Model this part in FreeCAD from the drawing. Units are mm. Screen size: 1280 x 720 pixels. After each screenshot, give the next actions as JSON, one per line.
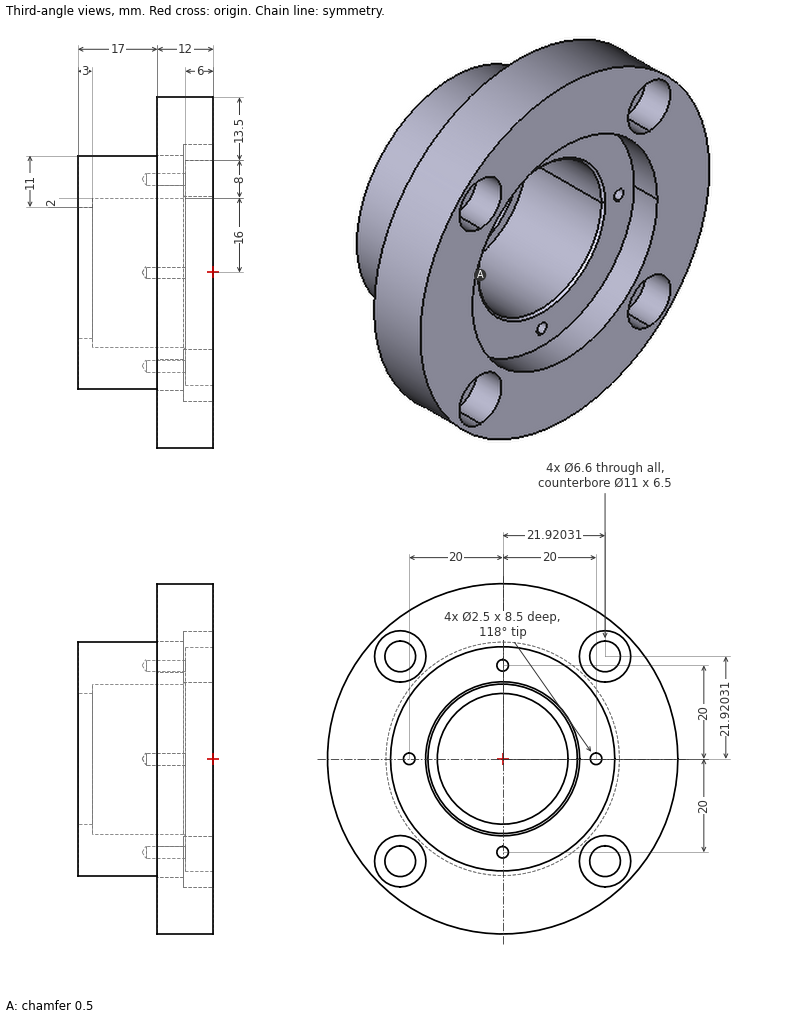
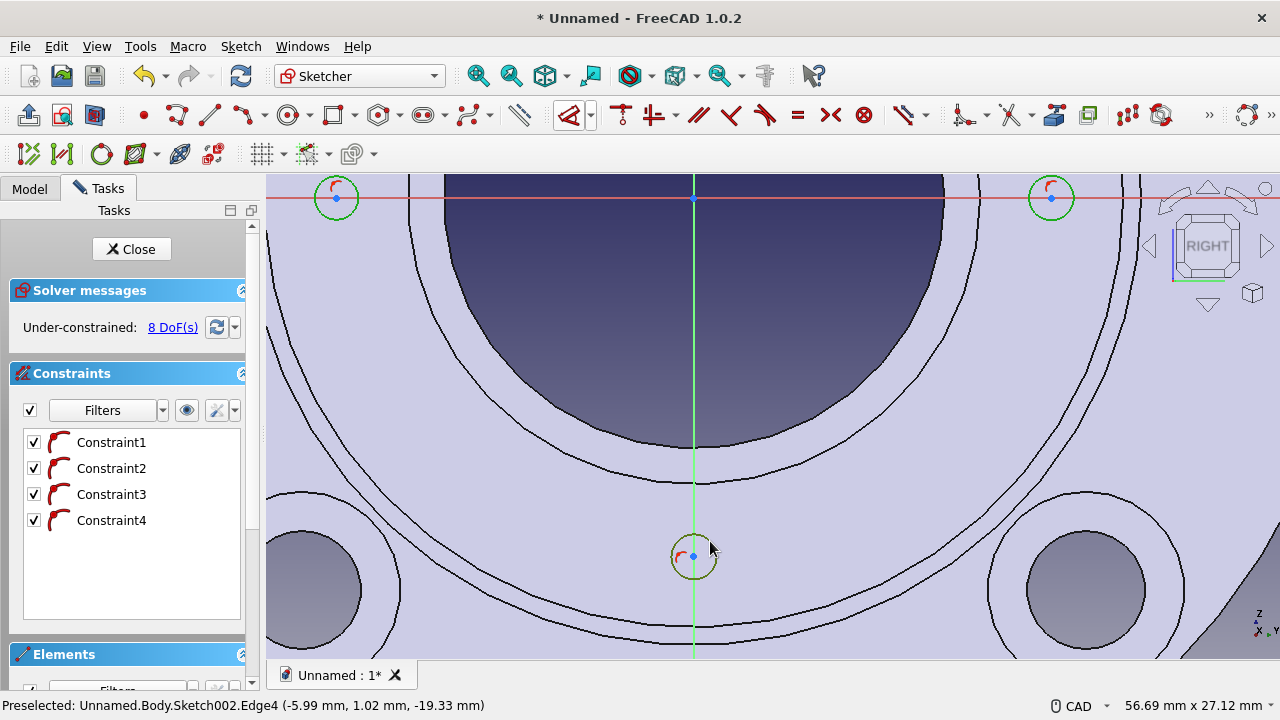
{"action": "key", "text": "e"}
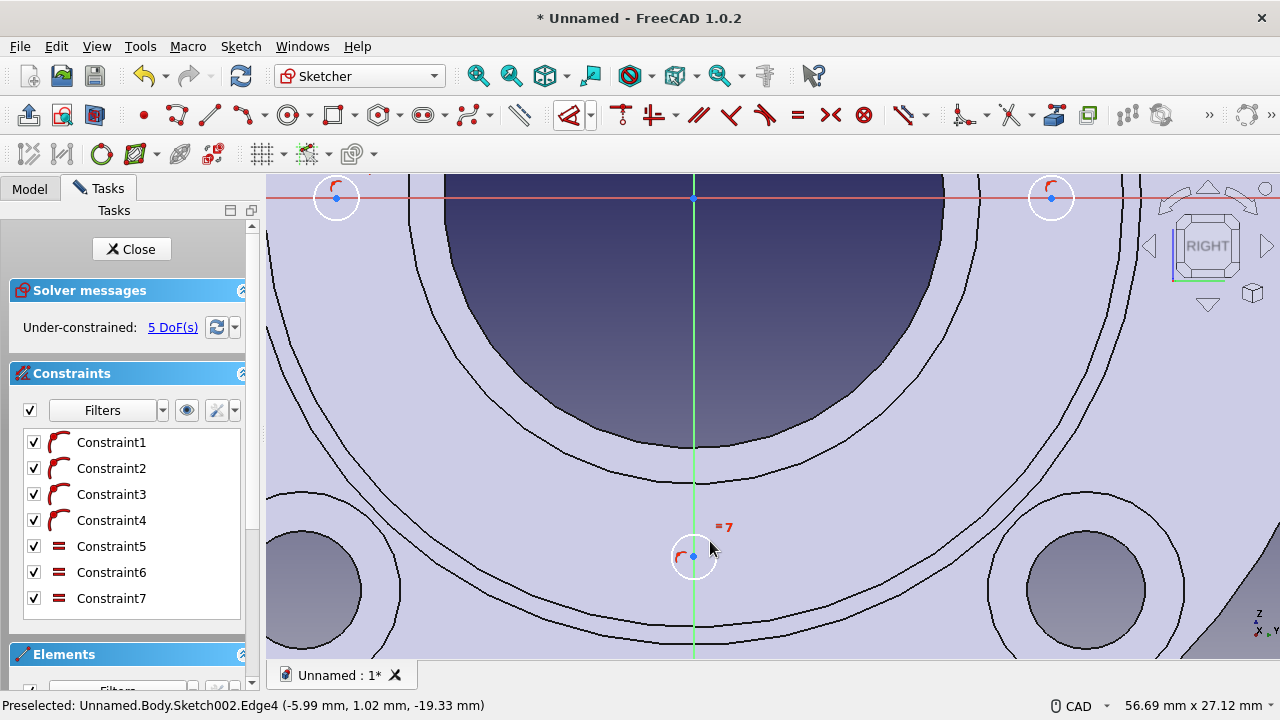
{"action": "left_click", "coordinate": [1036, 214]}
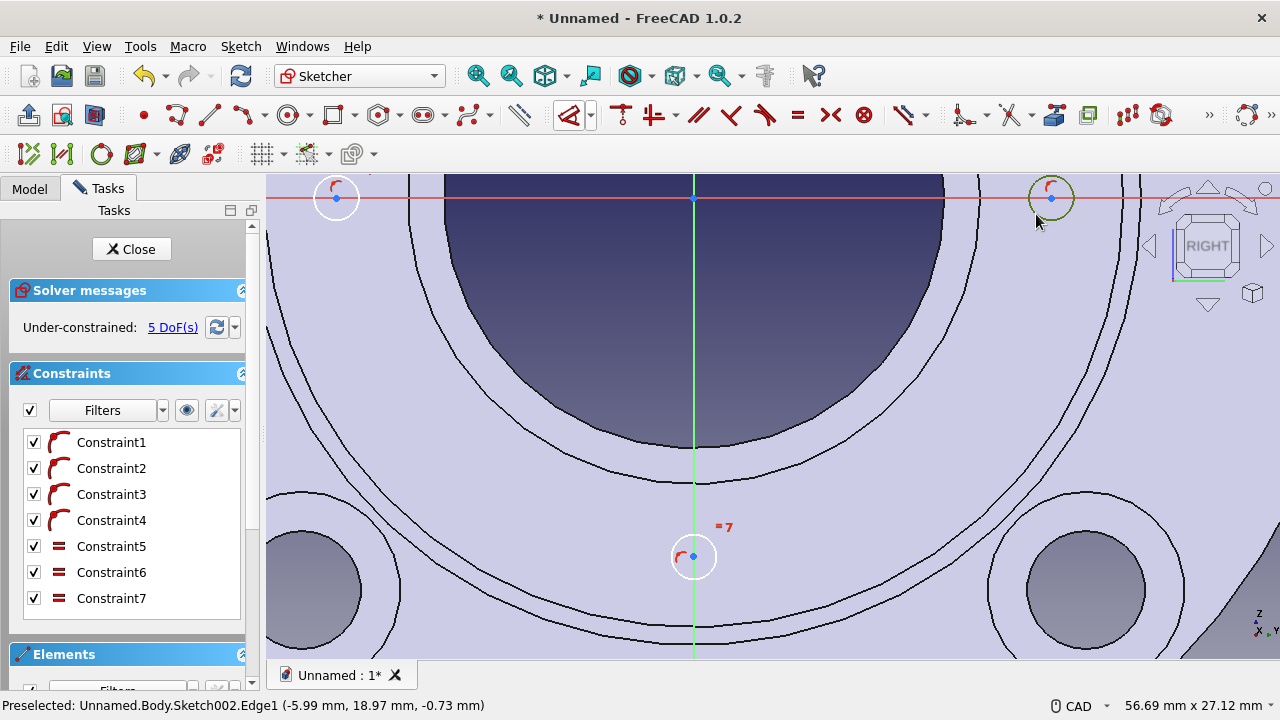
{"action": "key", "text": "k o"}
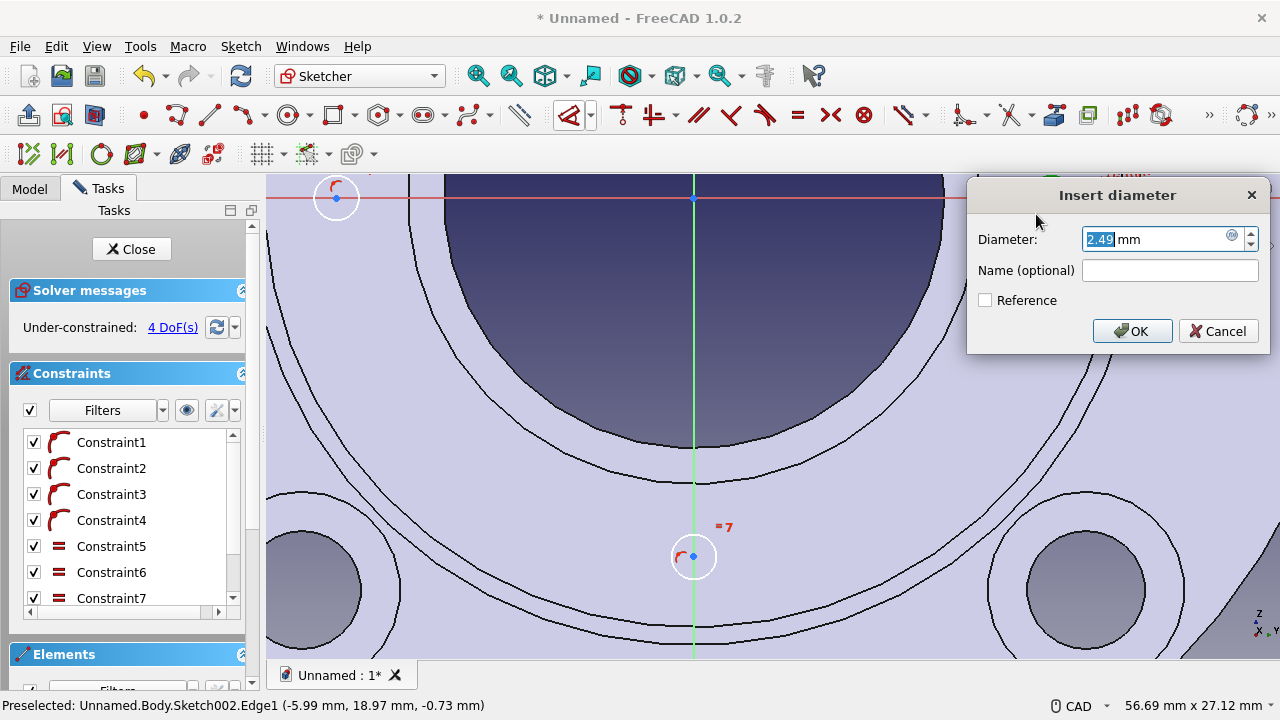
{"action": "type", "text": "2.5"}
{"action": "key", "text": "Return"}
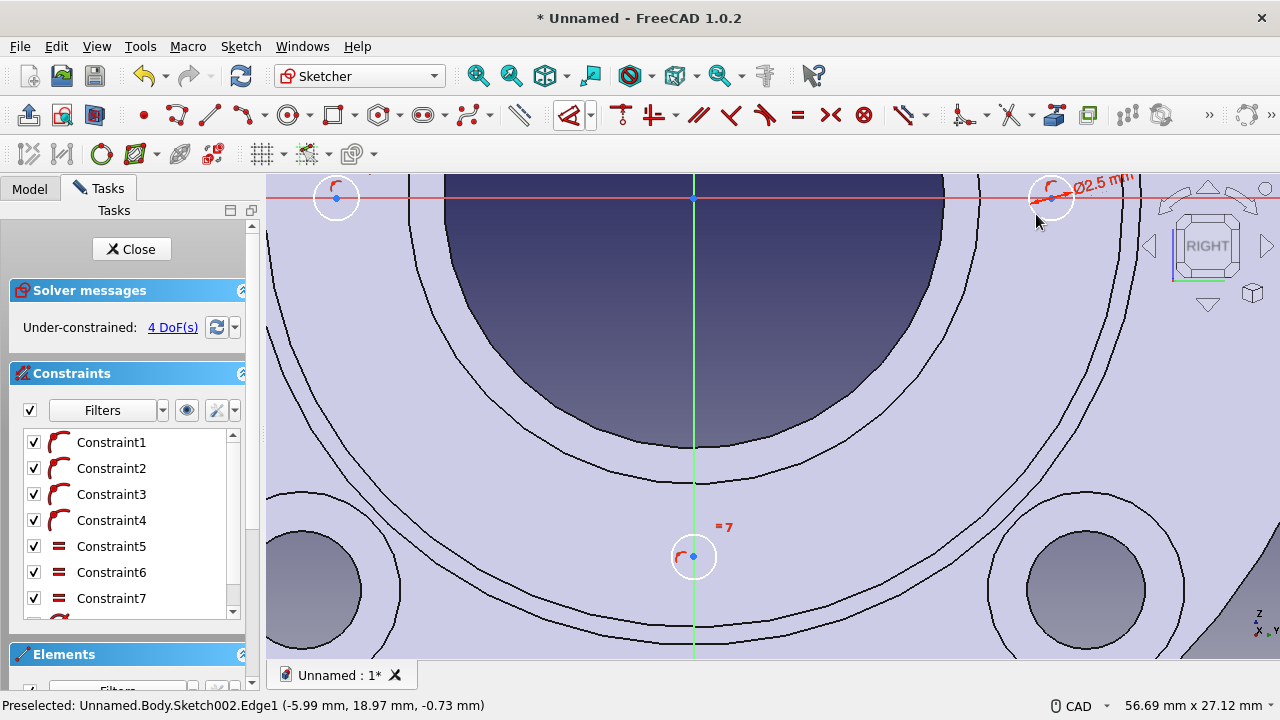
{"action": "scroll", "coordinate": [711, 544], "scroll_direction": "down", "scroll_amount": 5}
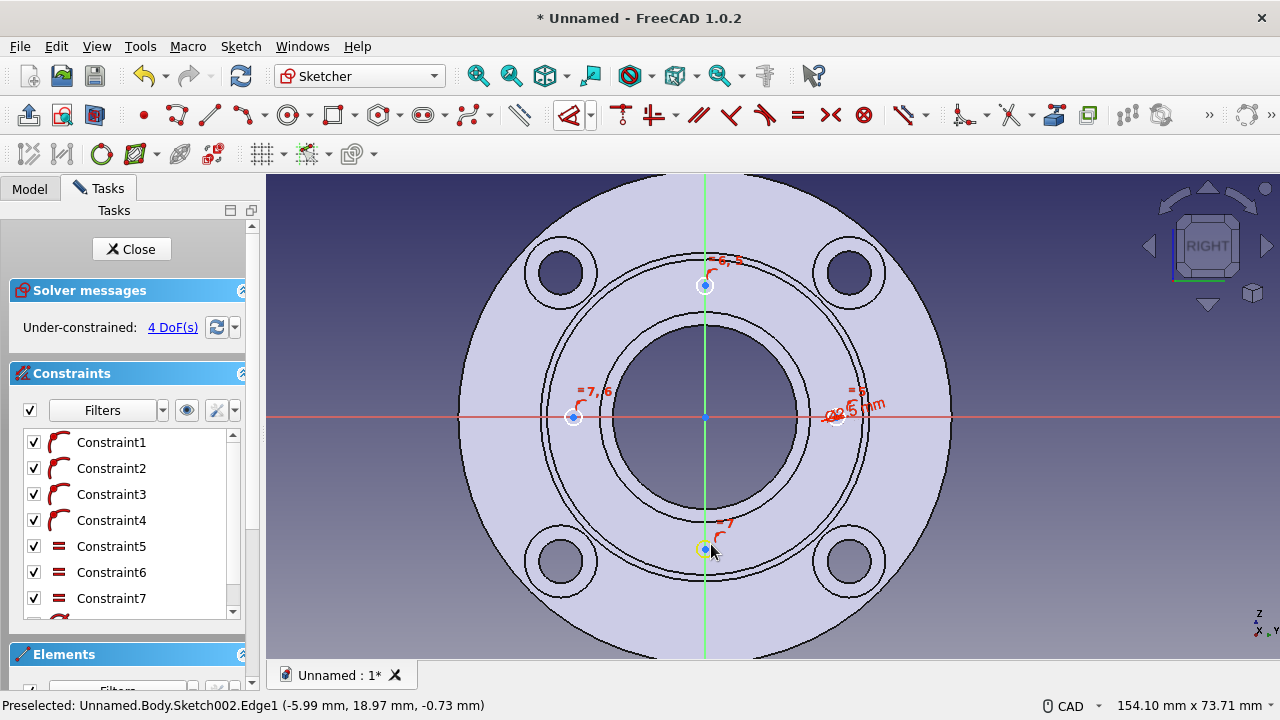
{"action": "left_click", "coordinate": [836, 417]}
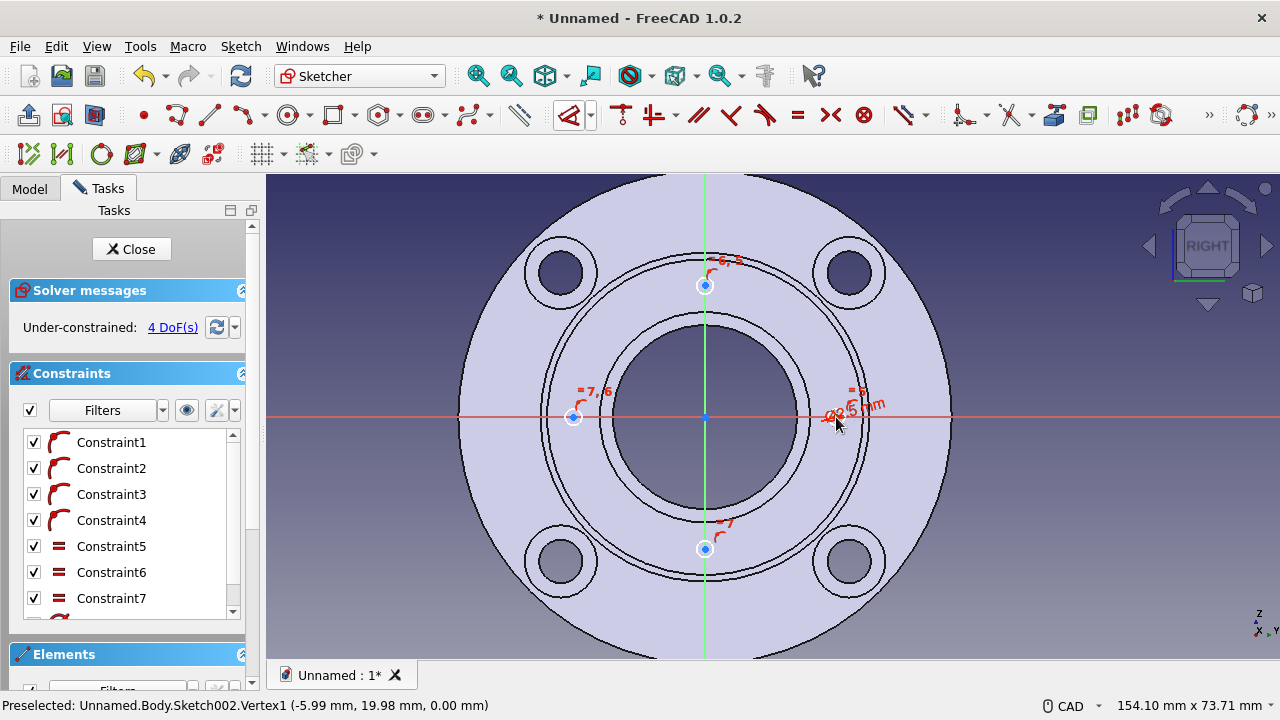
{"action": "left_click", "coordinate": [590, 116]}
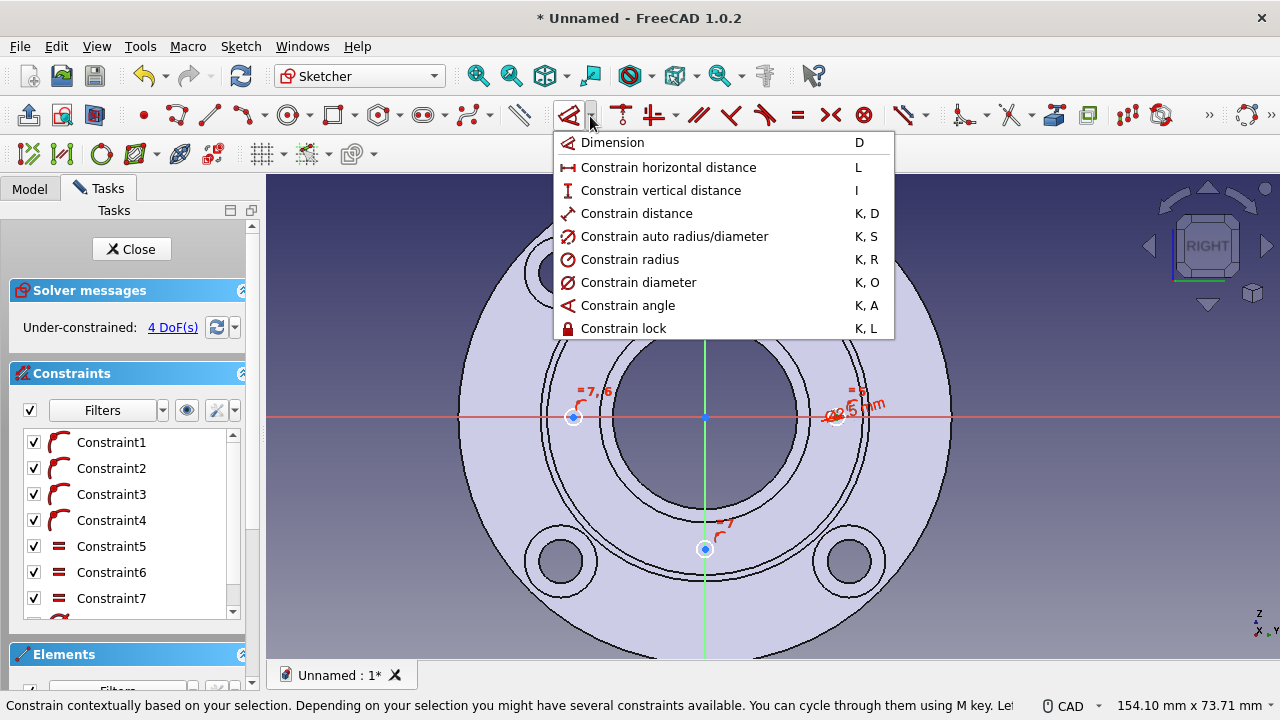
{"action": "left_click", "coordinate": [724, 168]}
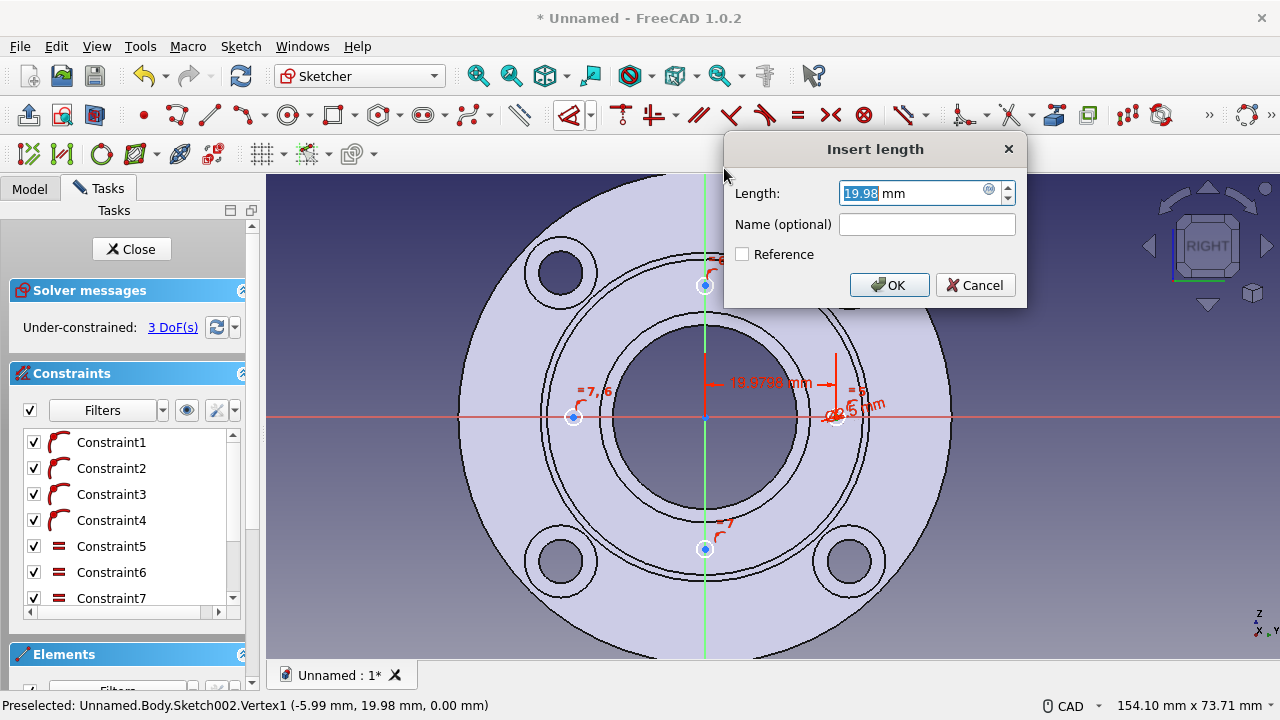
{"action": "type", "text": "20"}
{"action": "key", "text": "Return"}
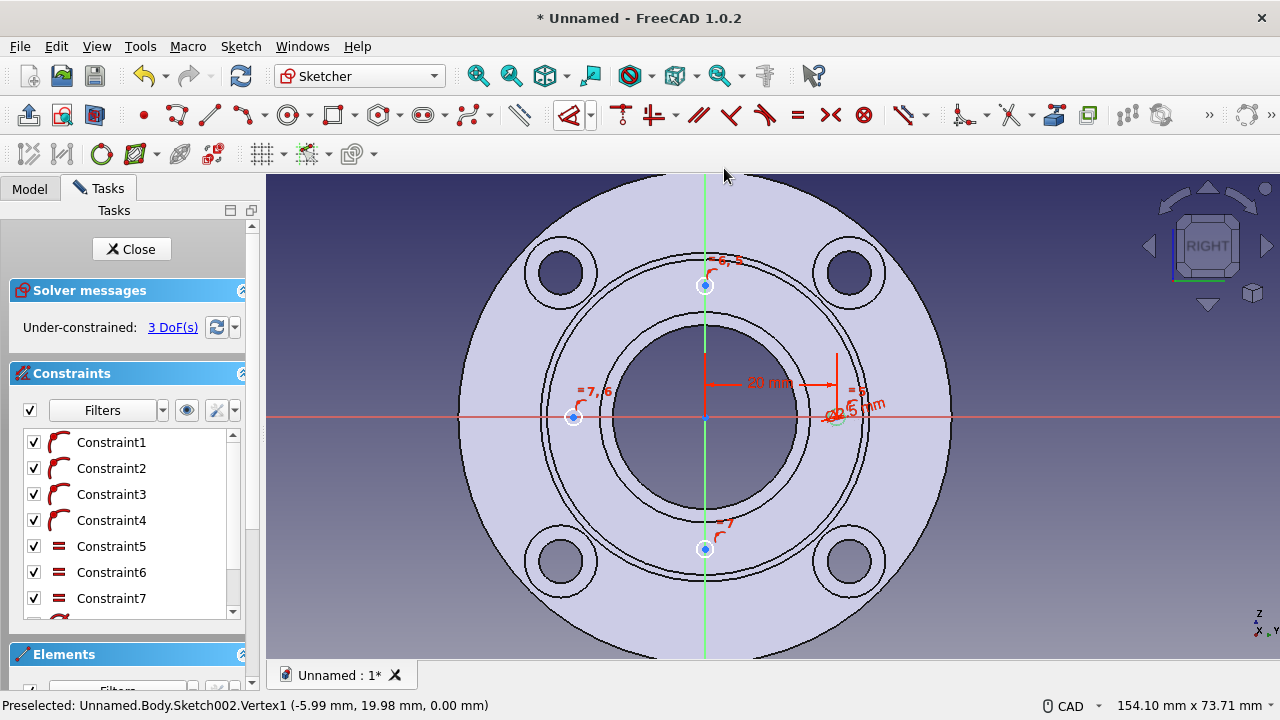
{"action": "left_click", "coordinate": [705, 286]}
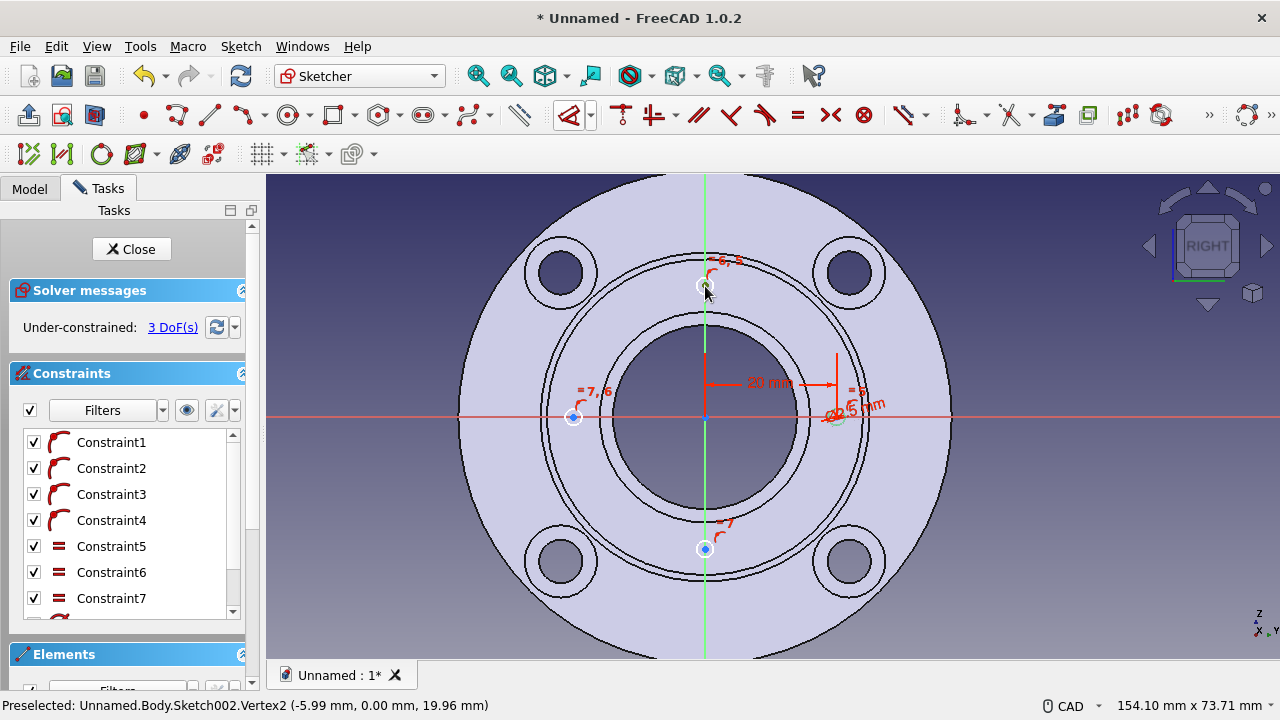
{"action": "left_click", "coordinate": [590, 116]}